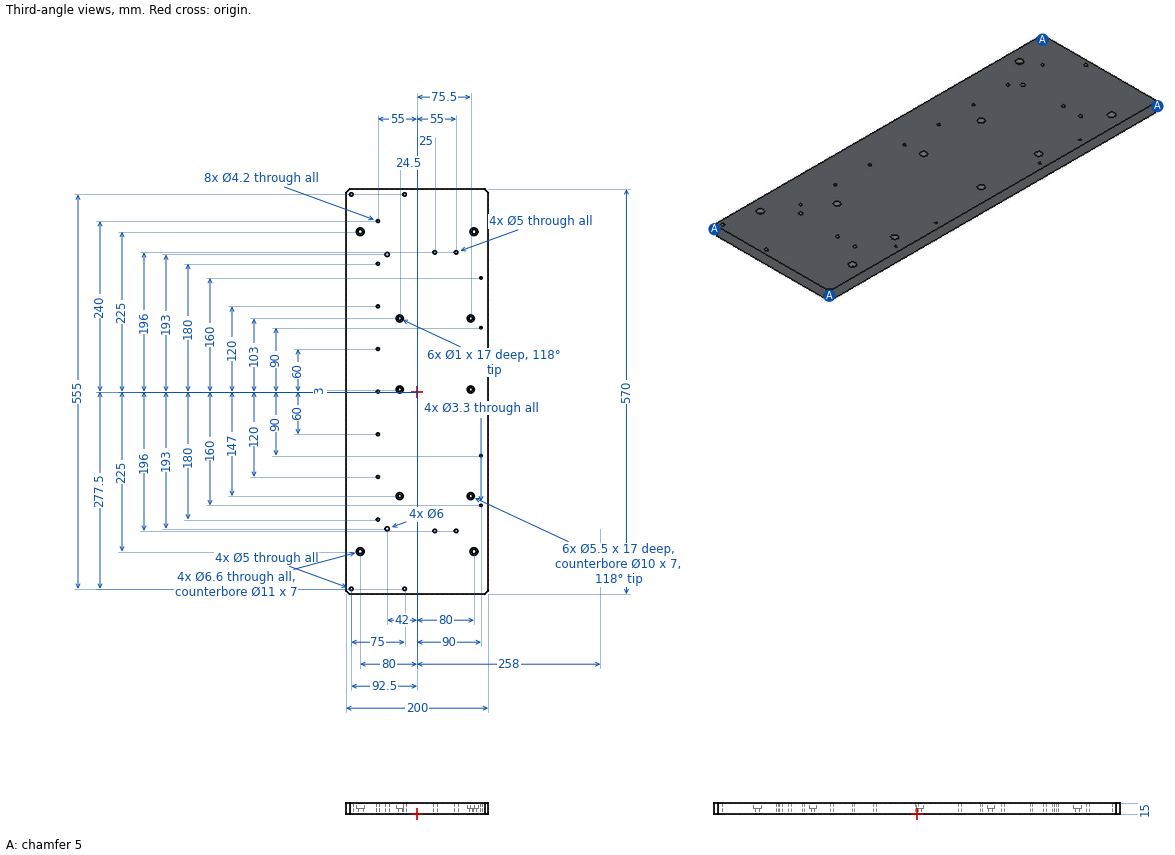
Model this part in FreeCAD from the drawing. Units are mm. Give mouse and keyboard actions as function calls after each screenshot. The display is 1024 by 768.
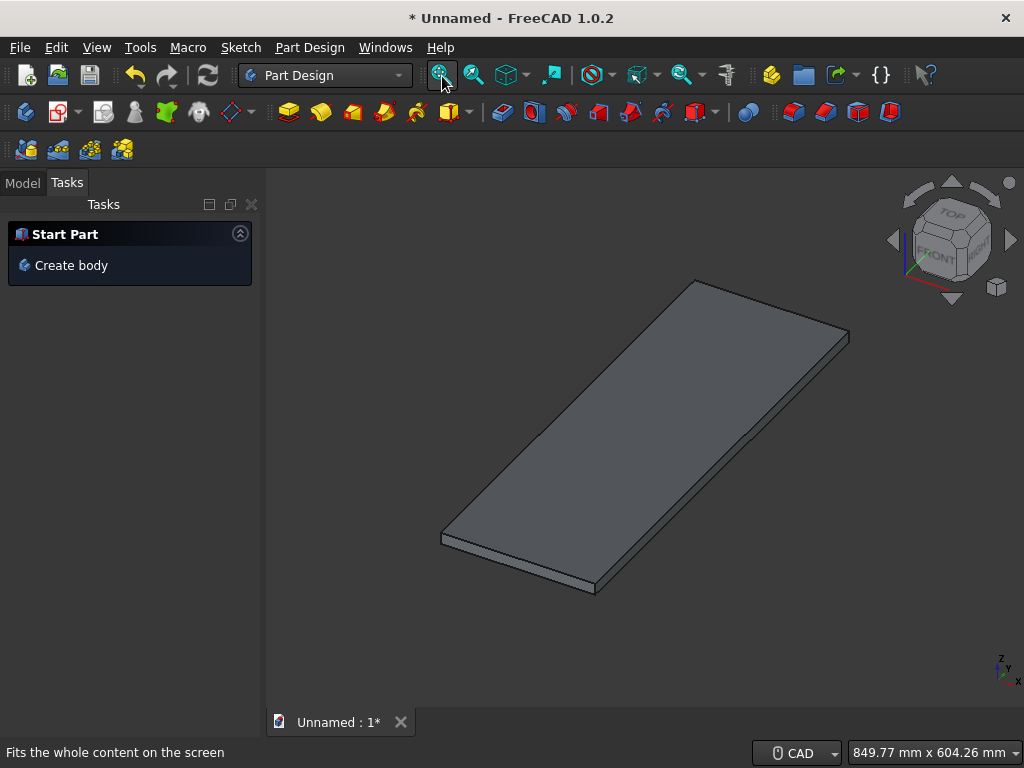
click(595, 589)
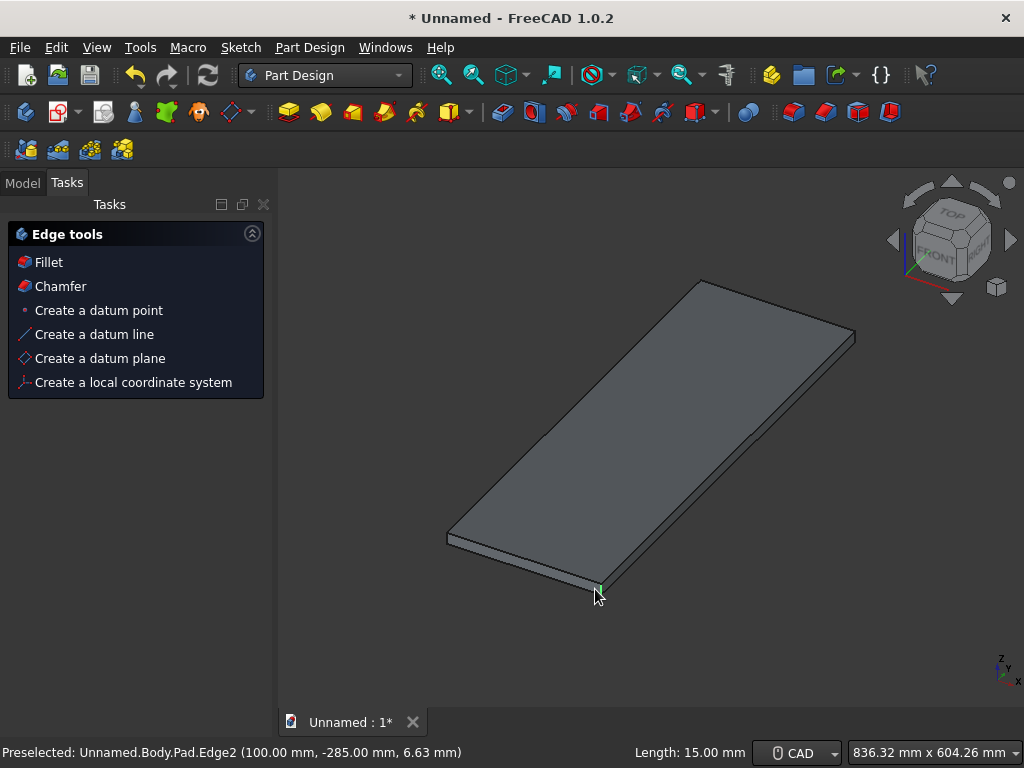
scroll(447, 537, up, 6)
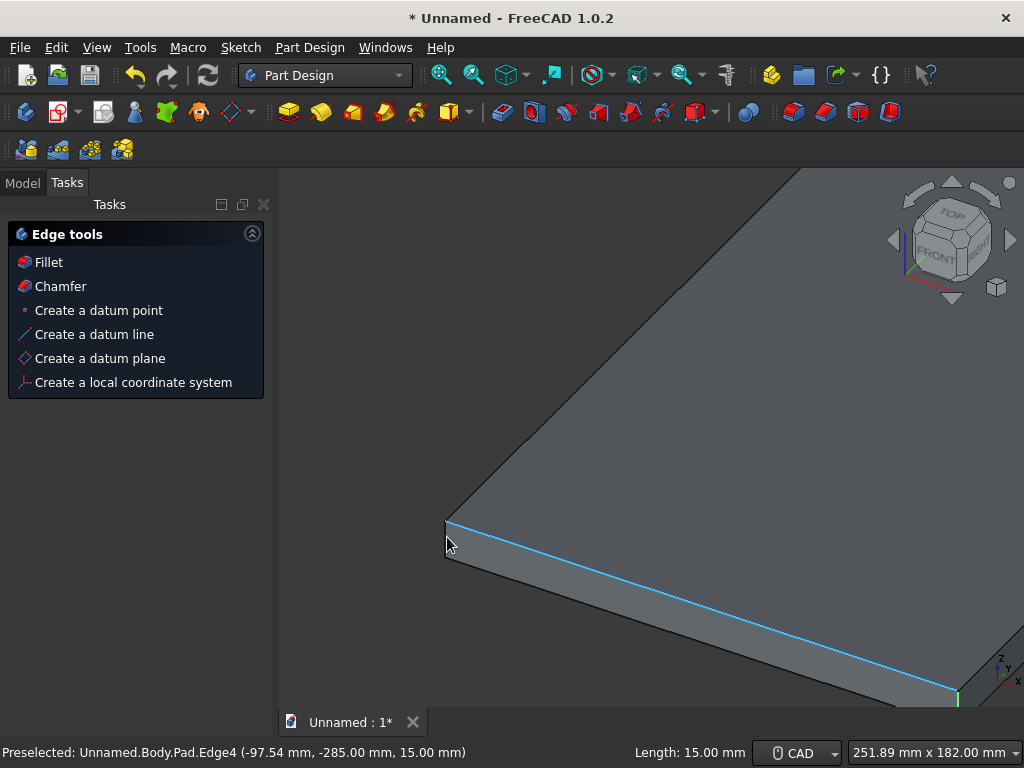
click(442, 76)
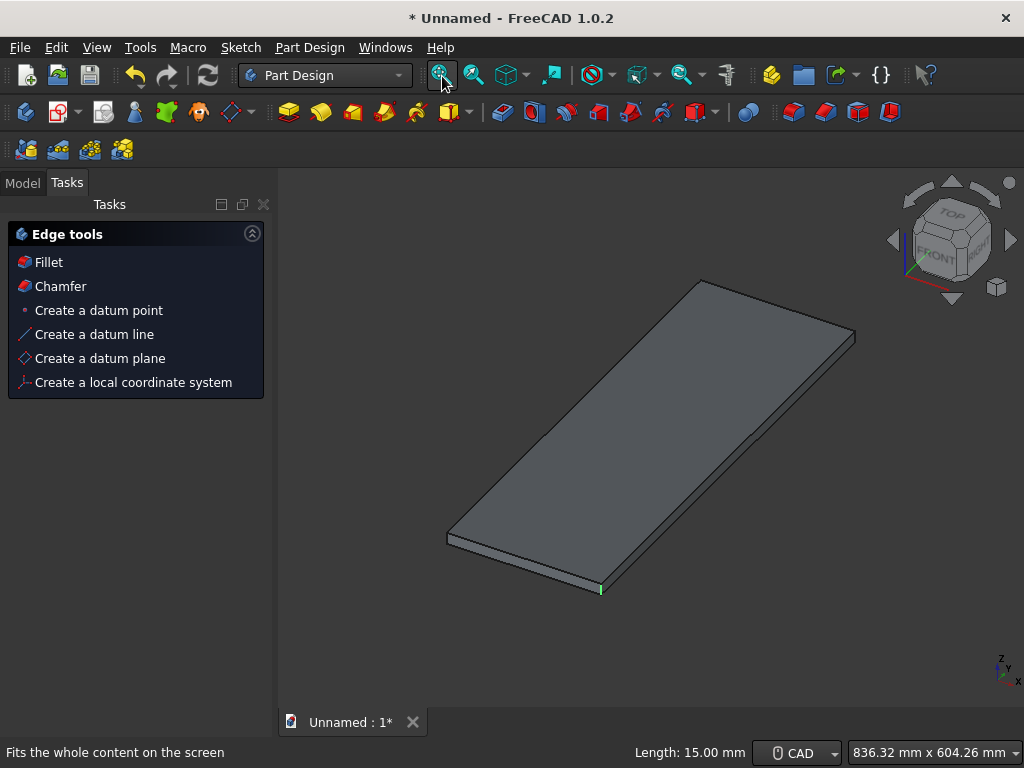
key(0)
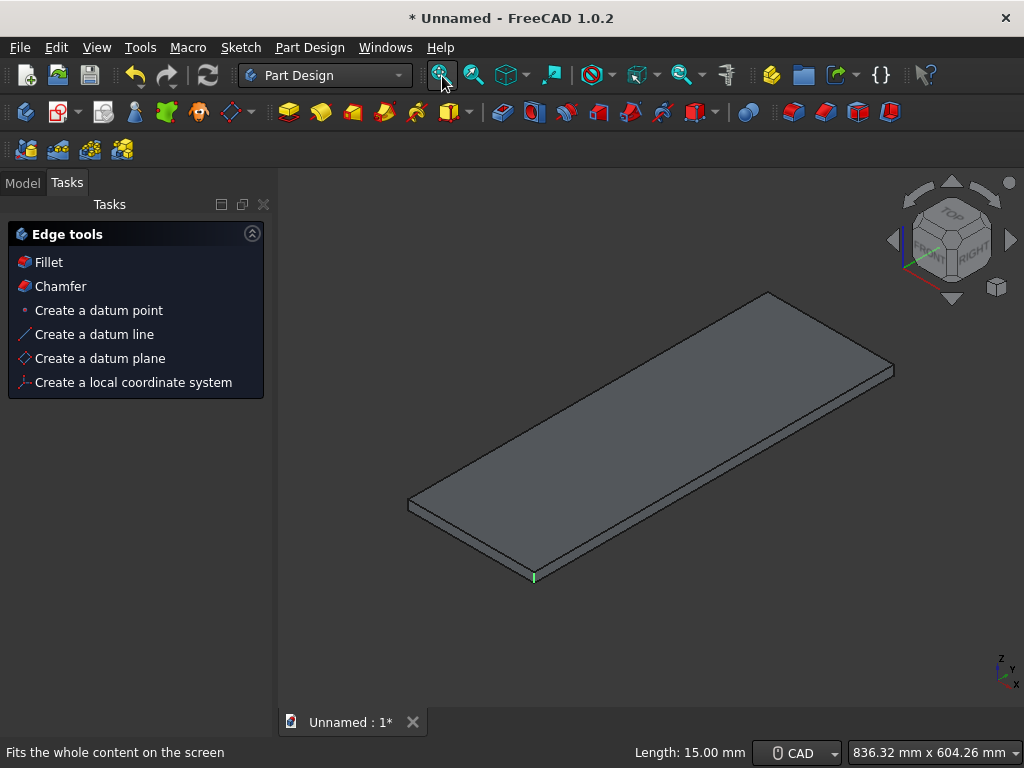
scroll(408, 504, up, 6)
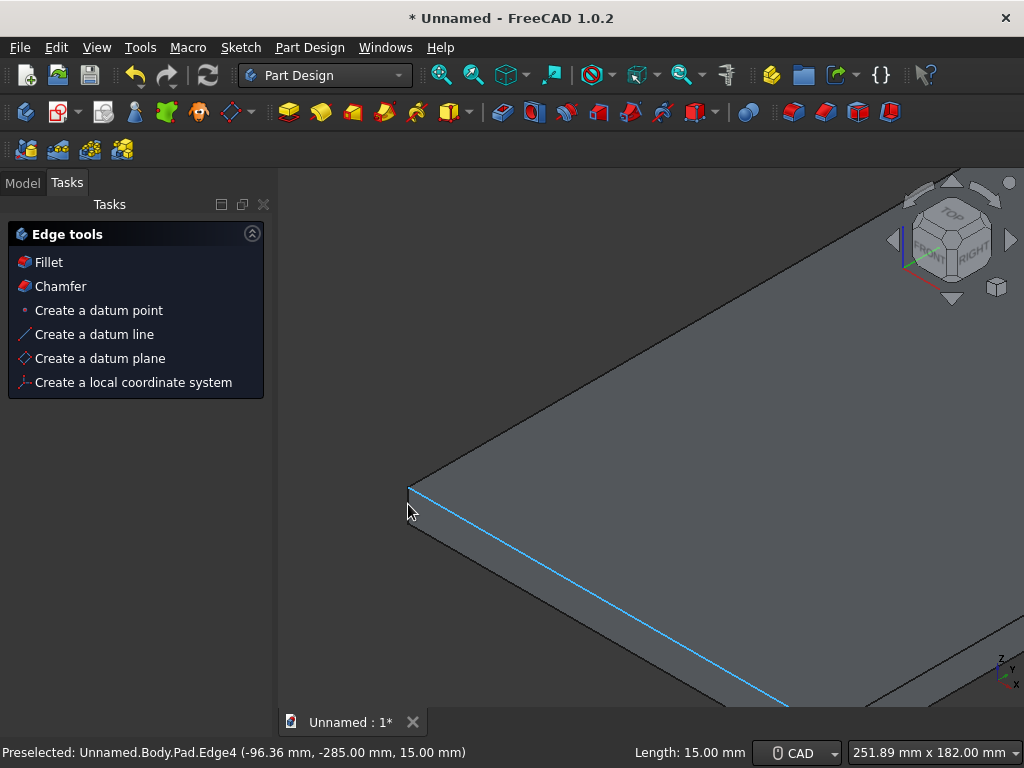
click(442, 76)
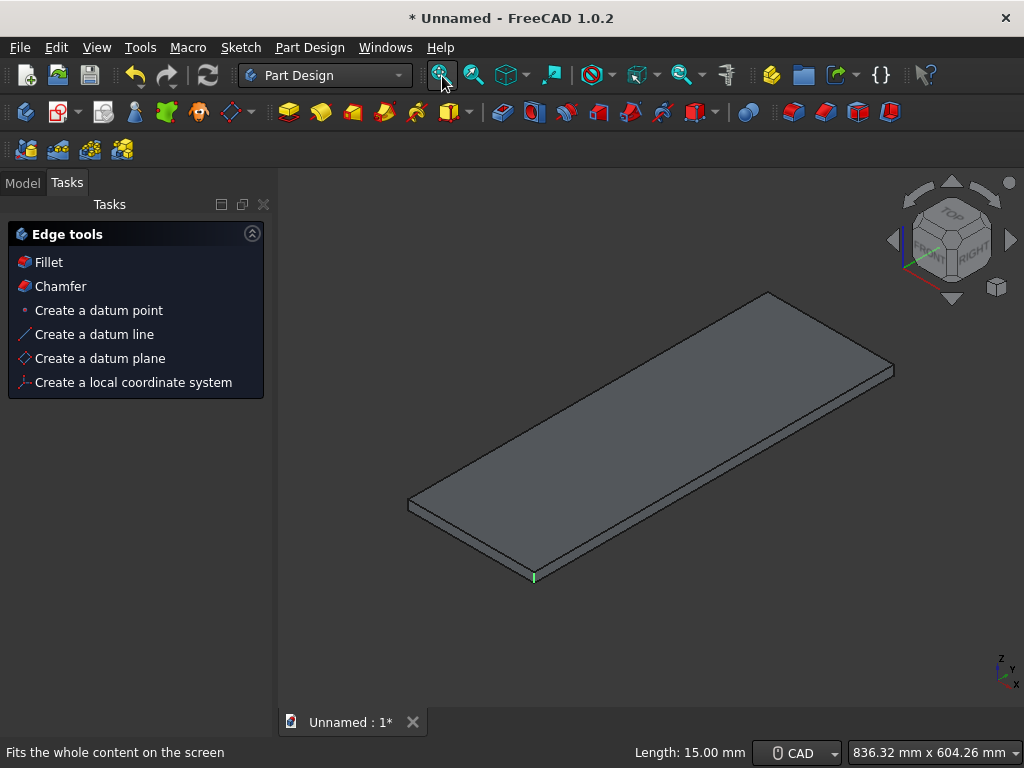
key(2)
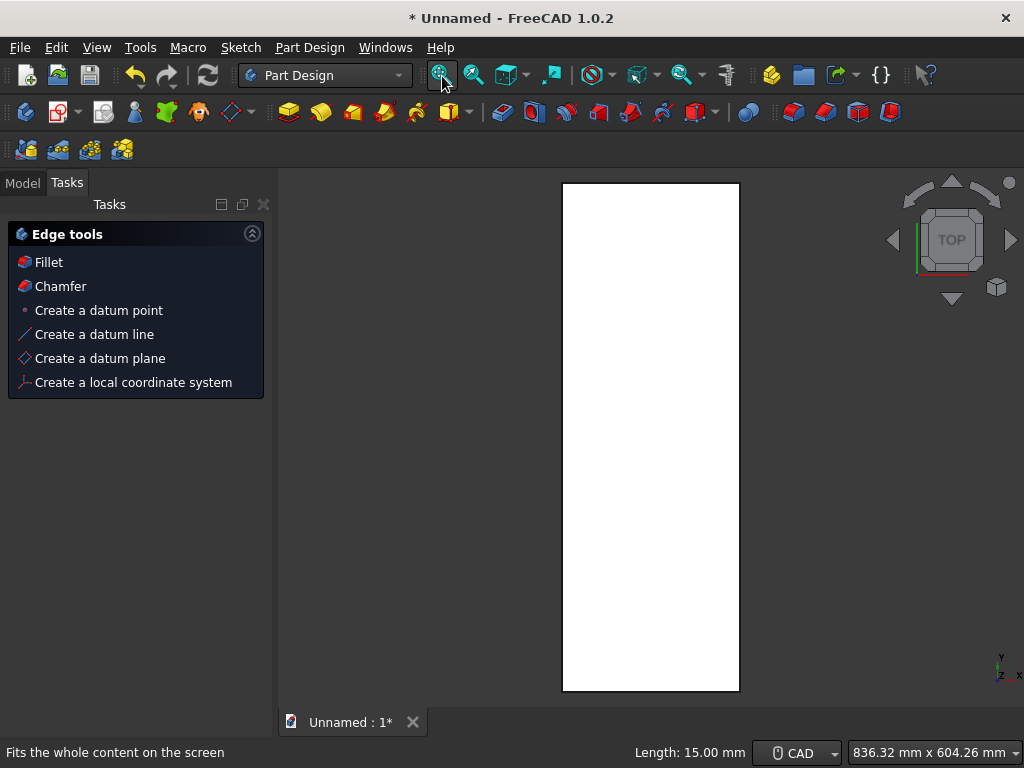
key(1)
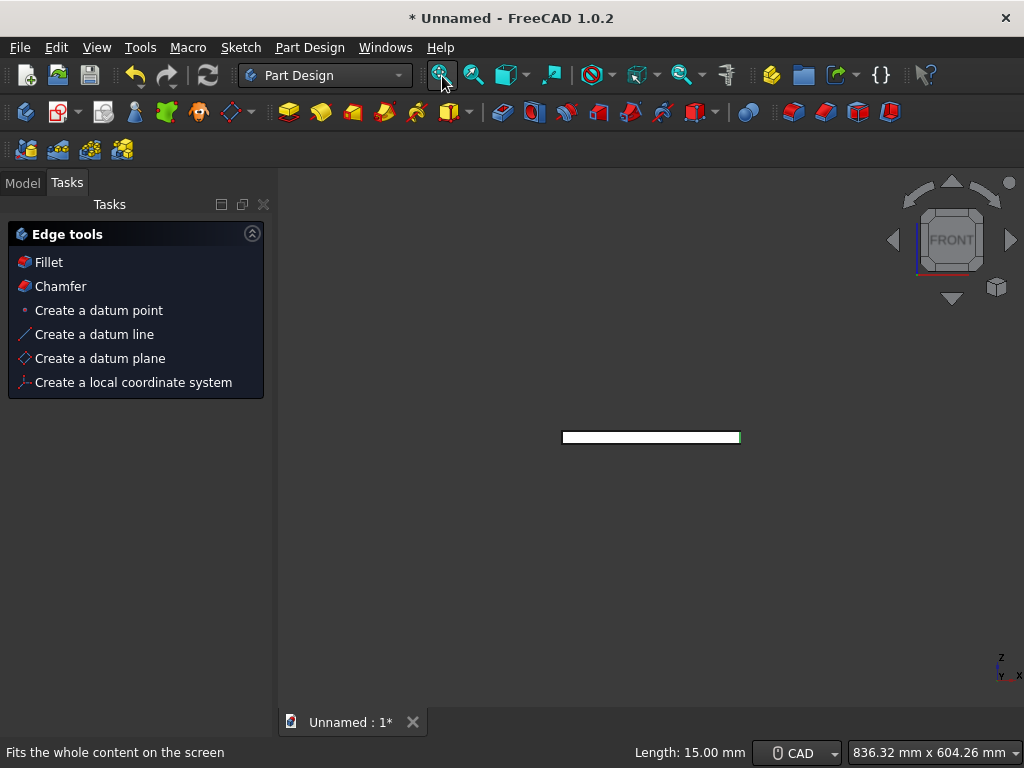
click(442, 76)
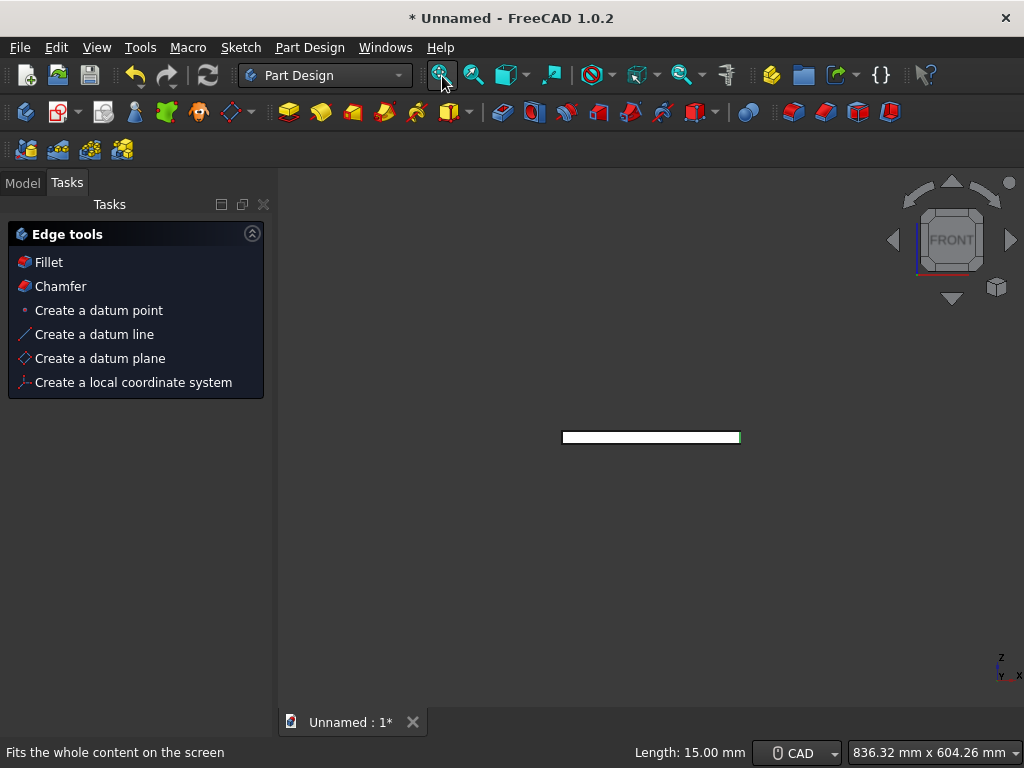
click(562, 437, ctrl)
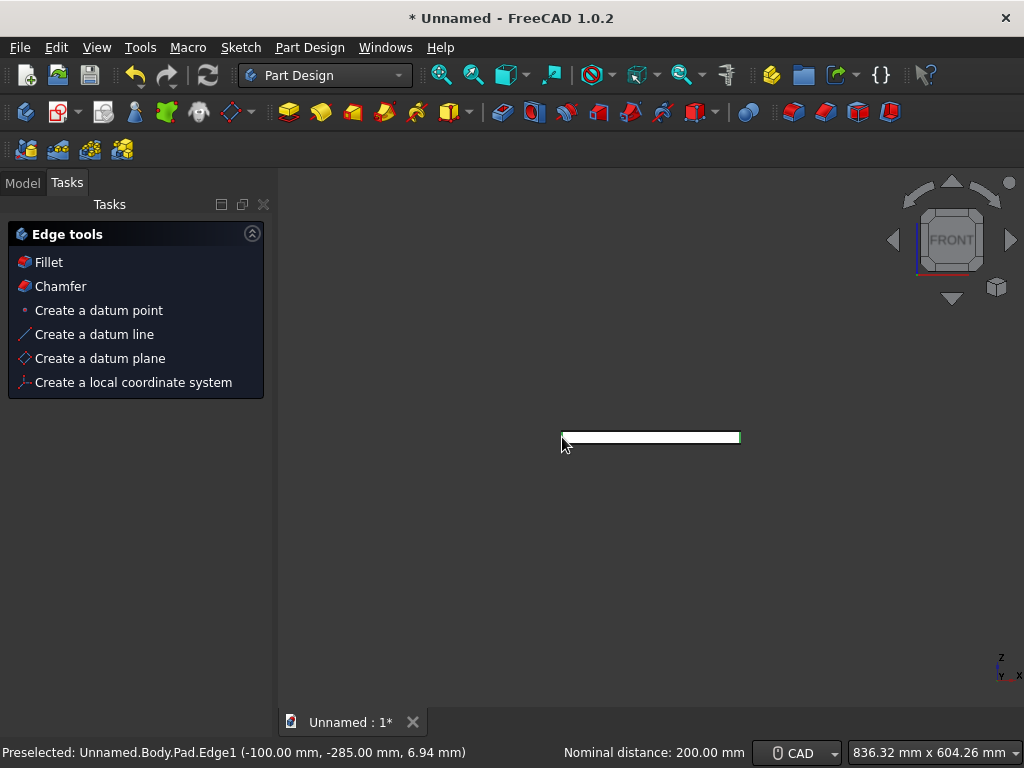
scroll(562, 437, up, 6)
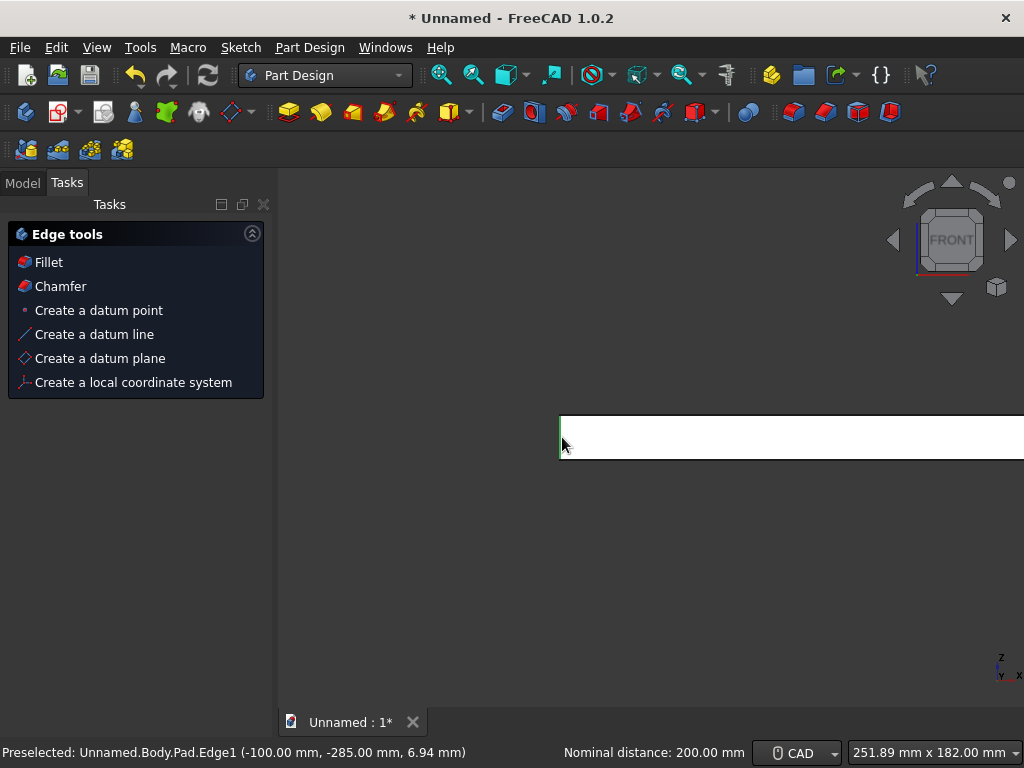
key(v)
key(f)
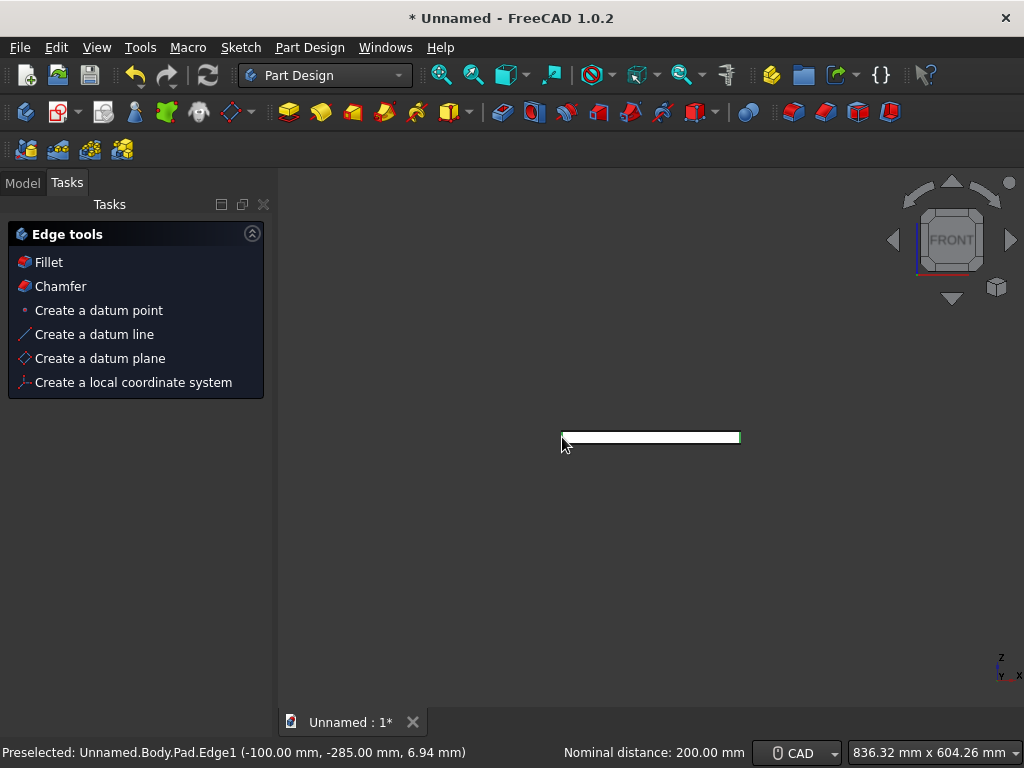
key(3)